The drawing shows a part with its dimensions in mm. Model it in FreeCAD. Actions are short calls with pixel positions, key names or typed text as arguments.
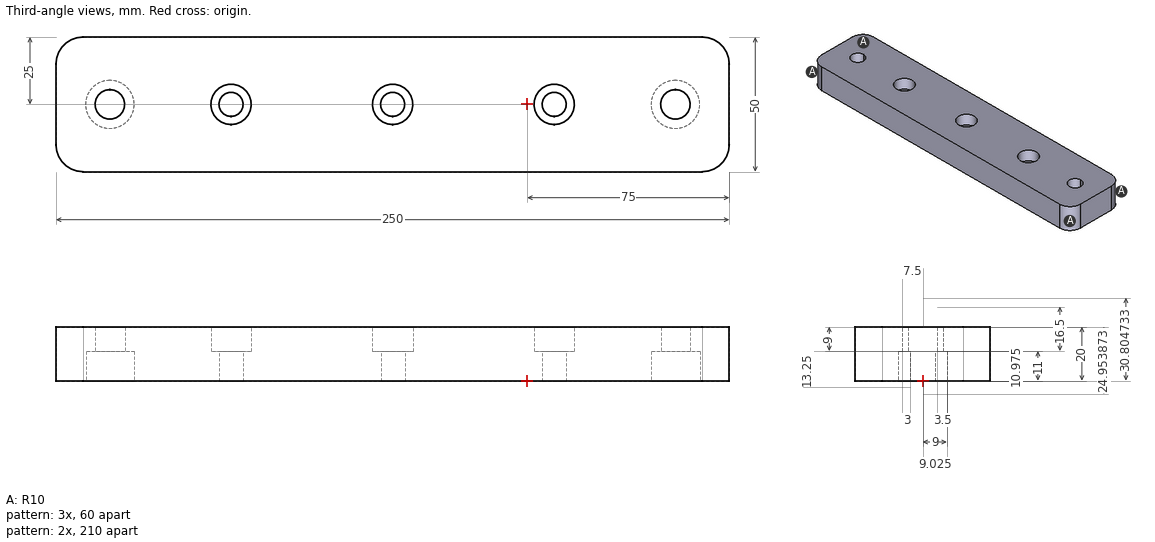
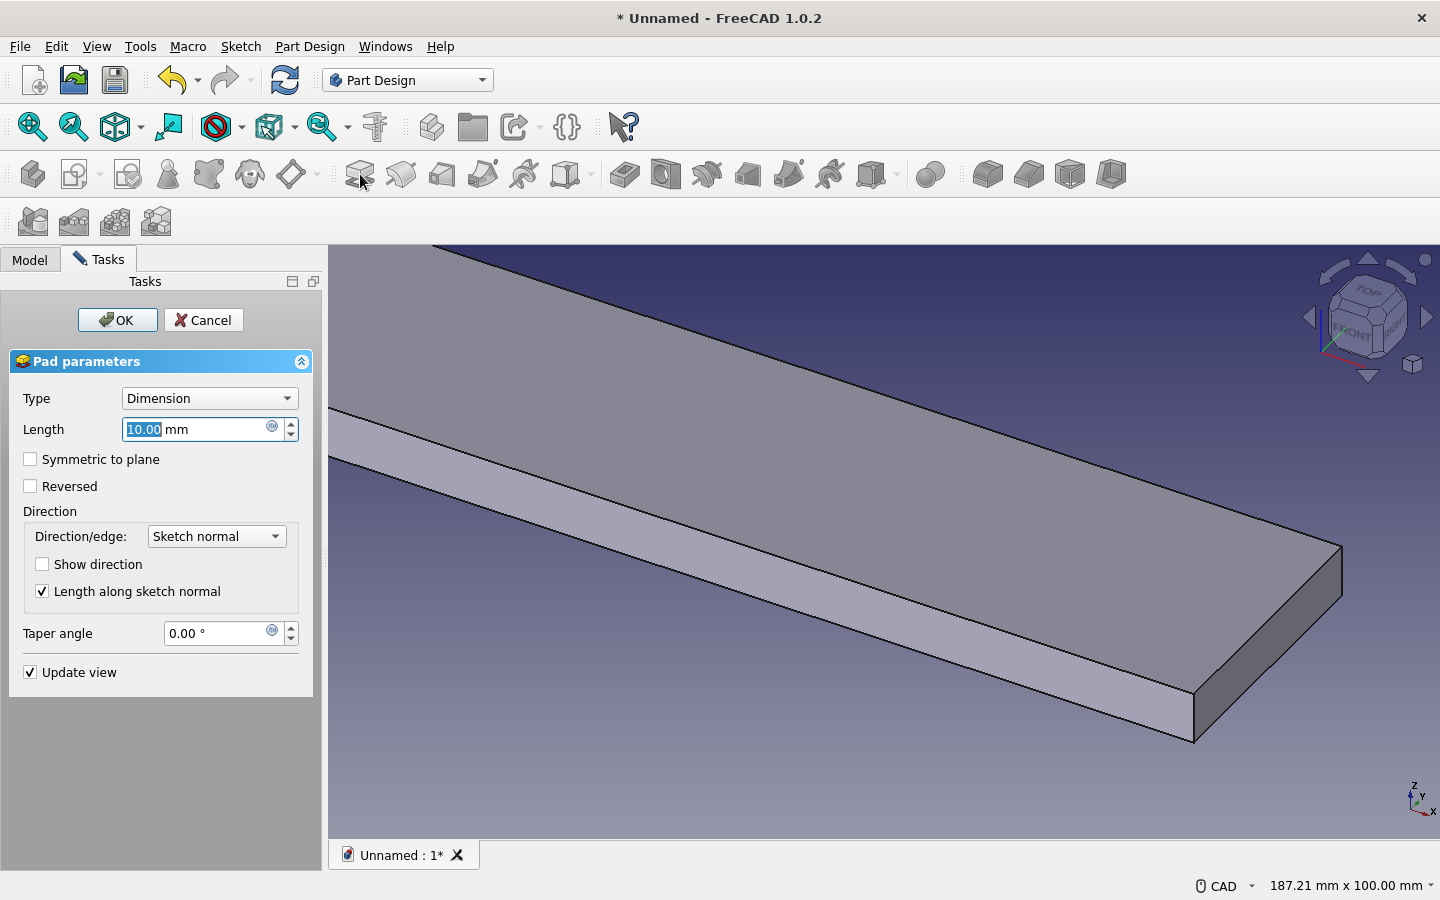
text(20)
key(Tab)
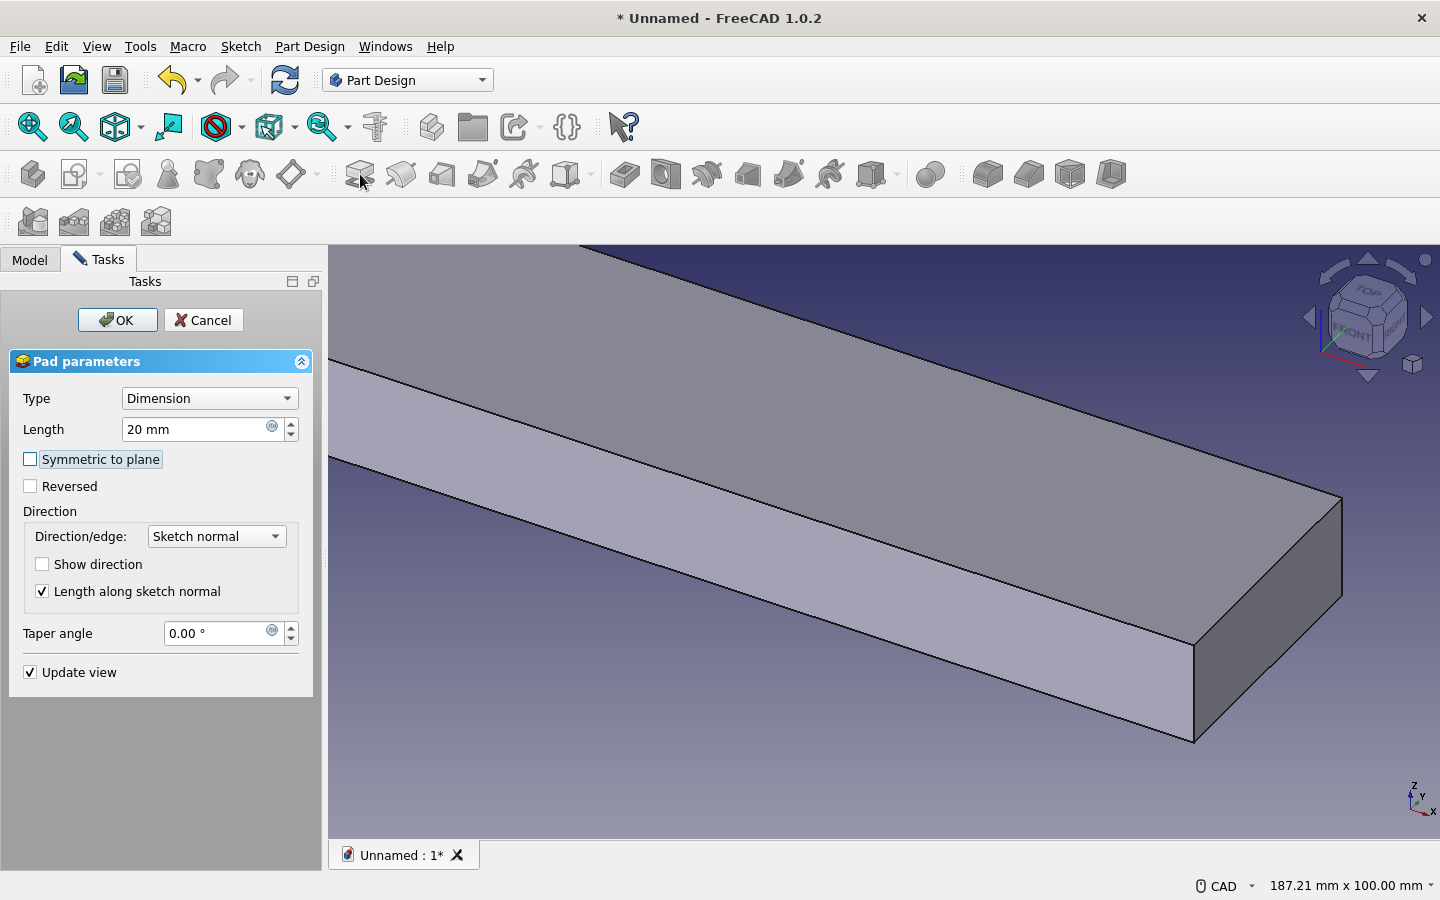
click(118, 320)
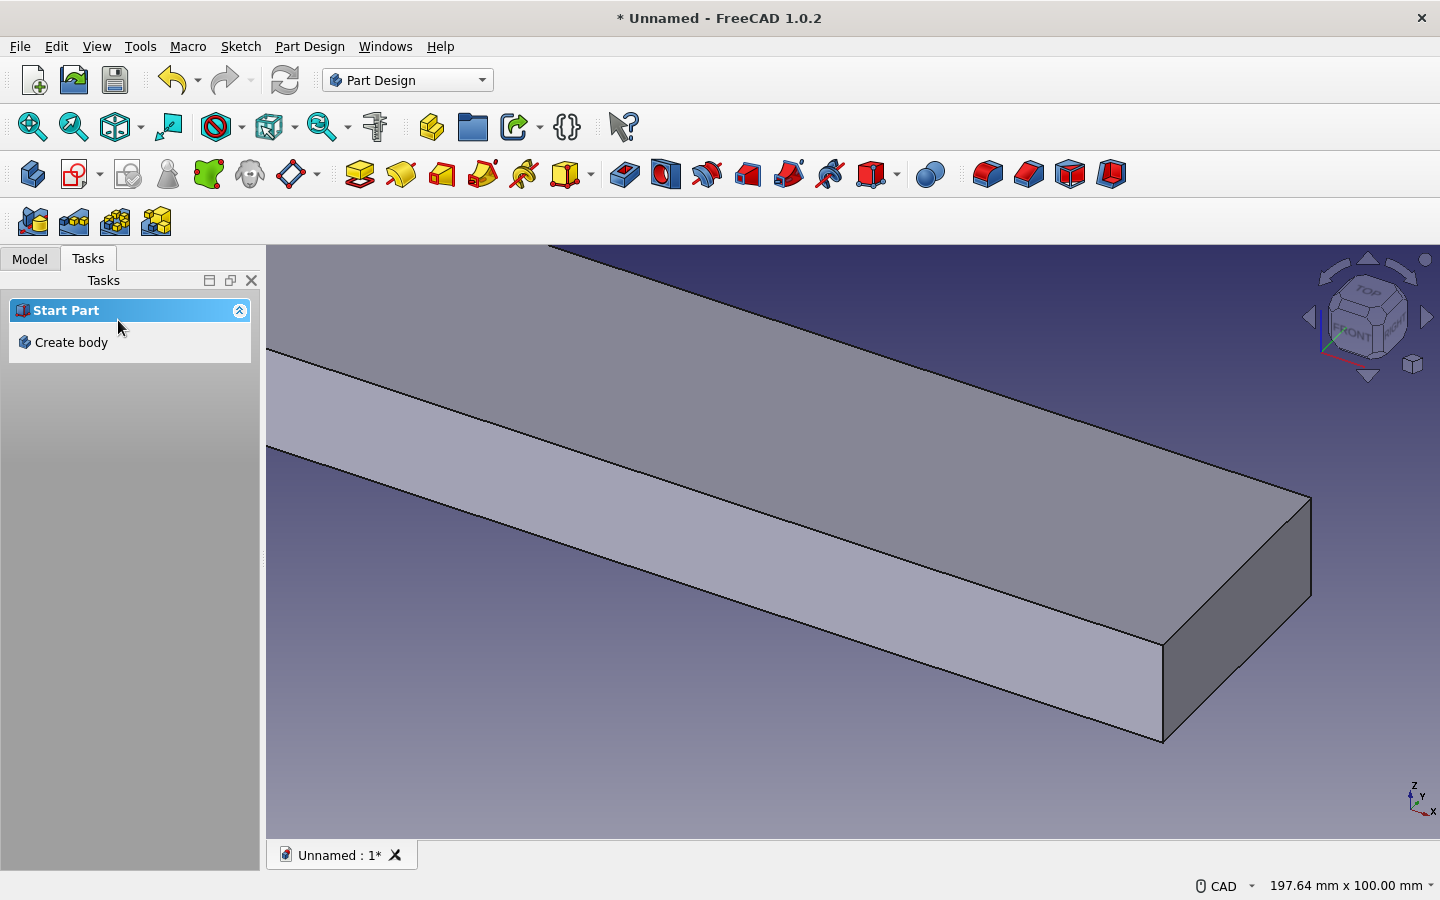
key(v)
key(f)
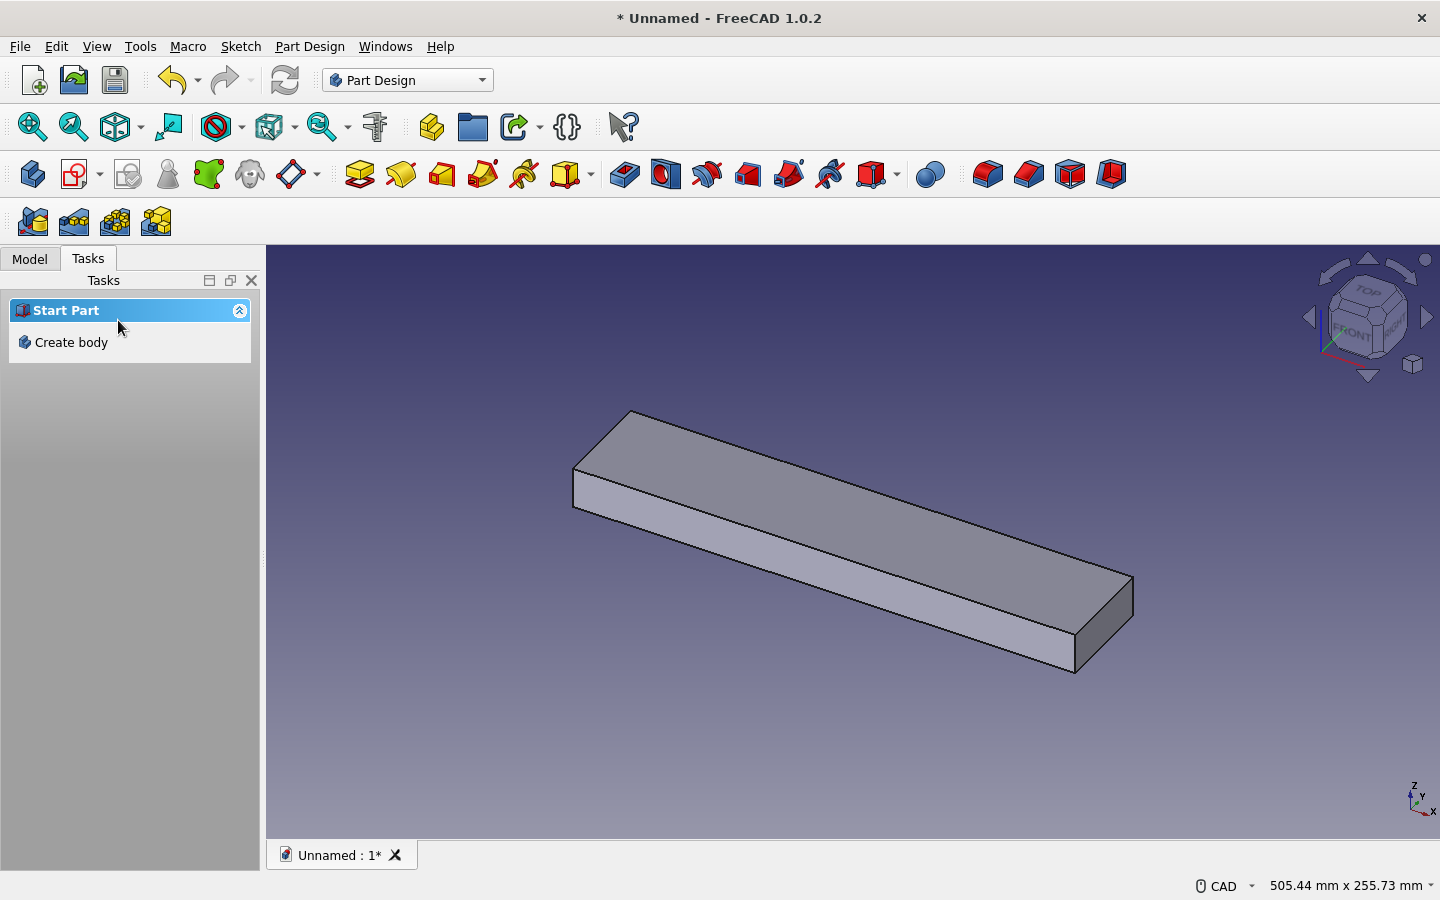
click(1075, 653)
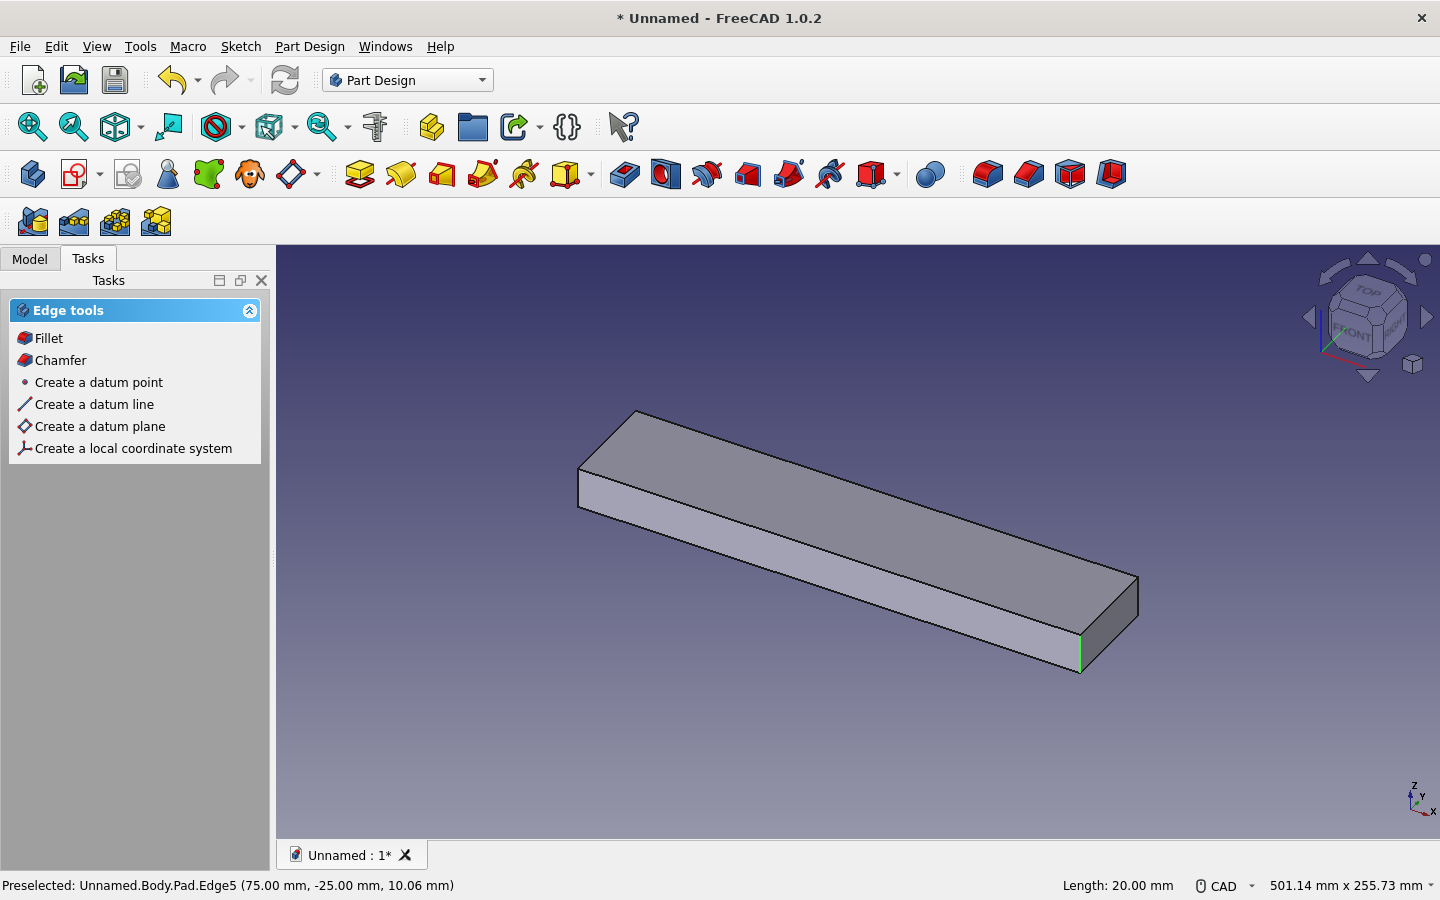
key(0)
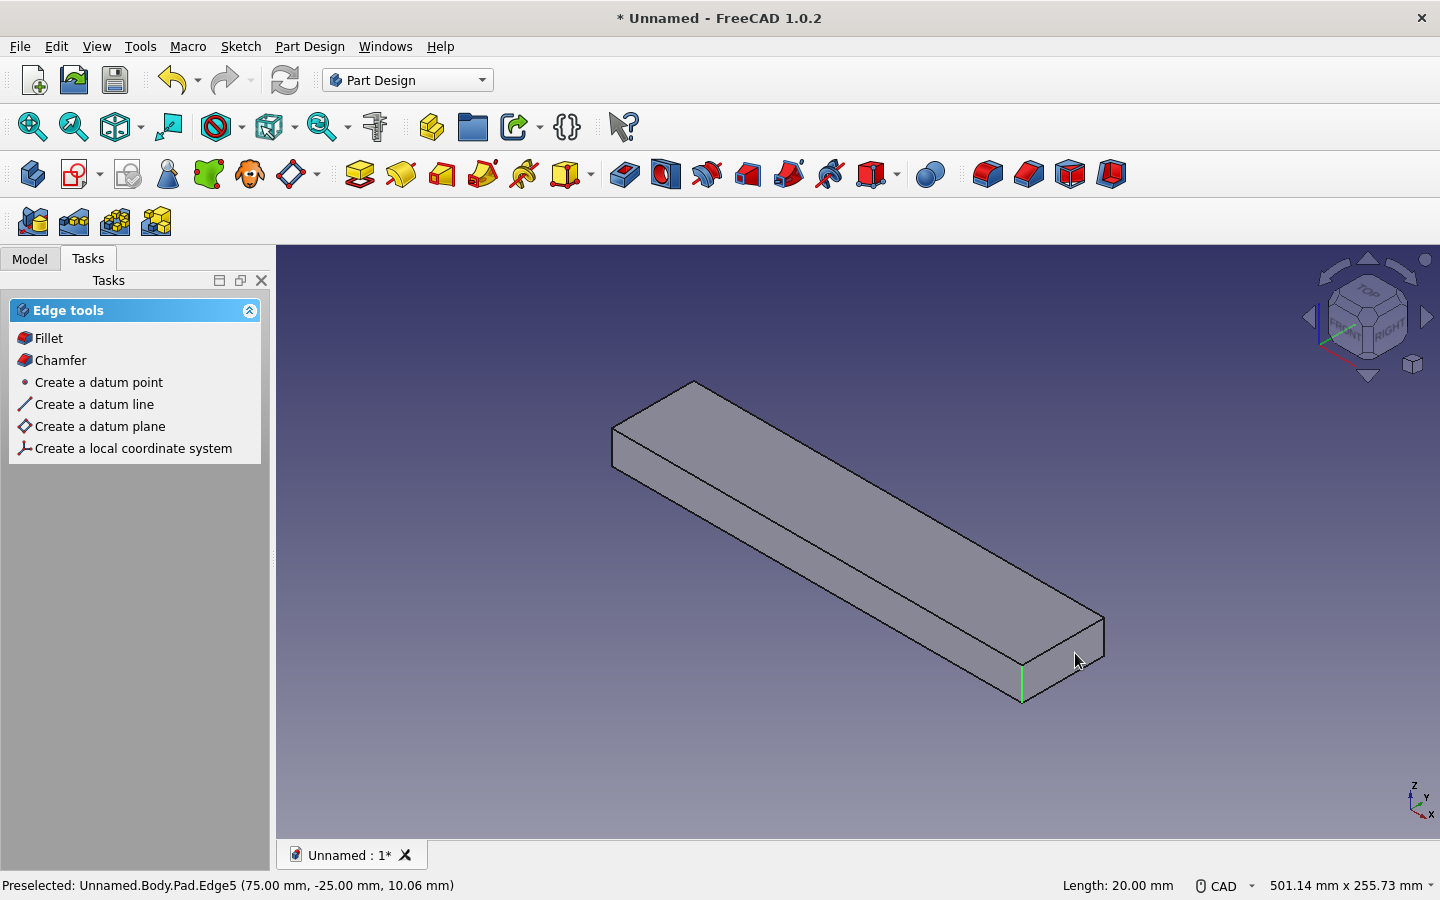
key(2)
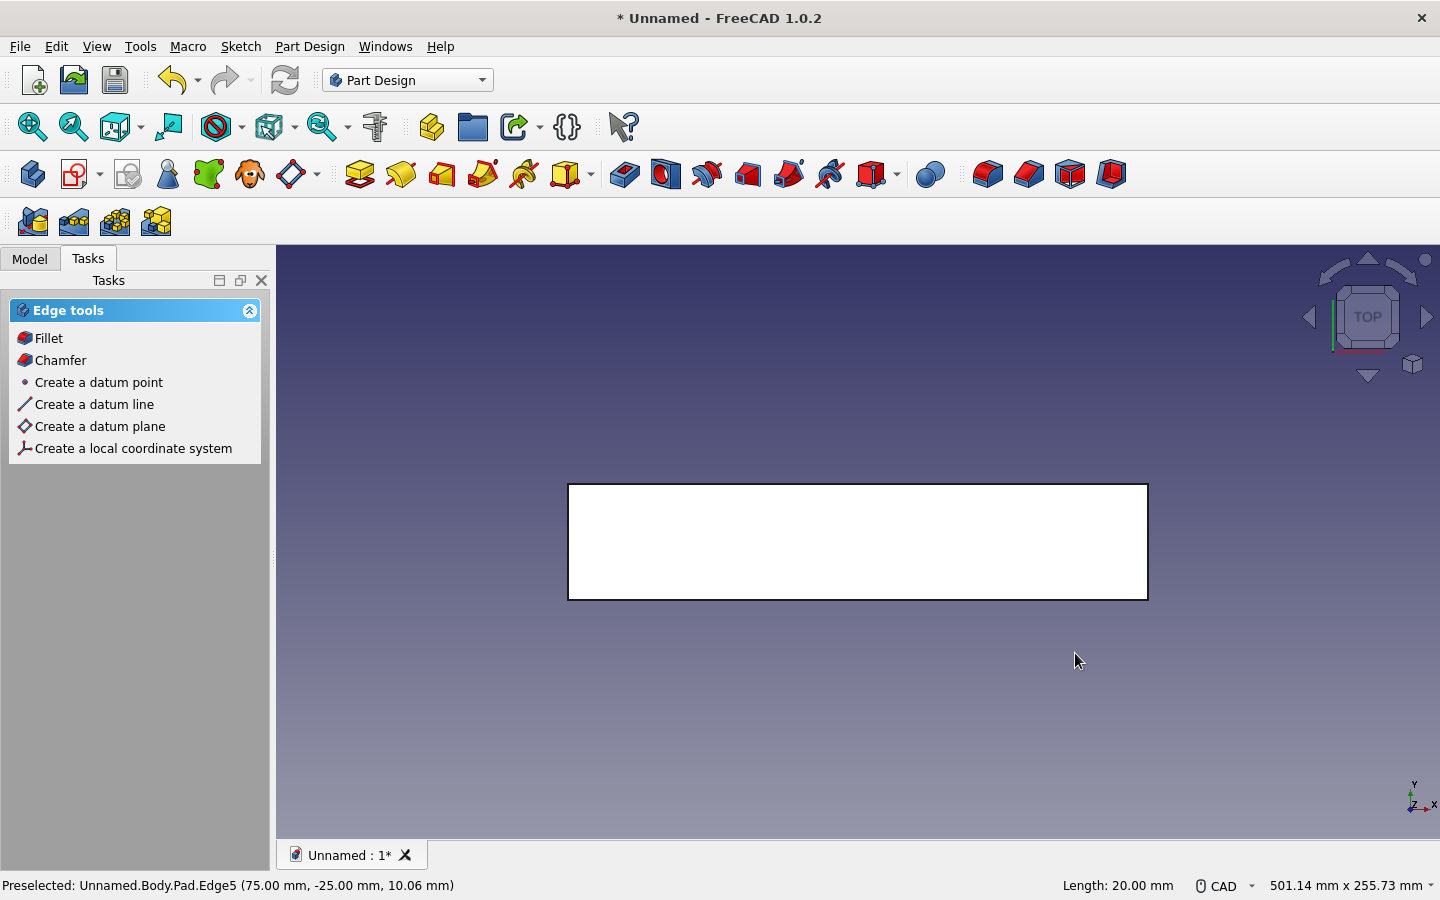
key(1)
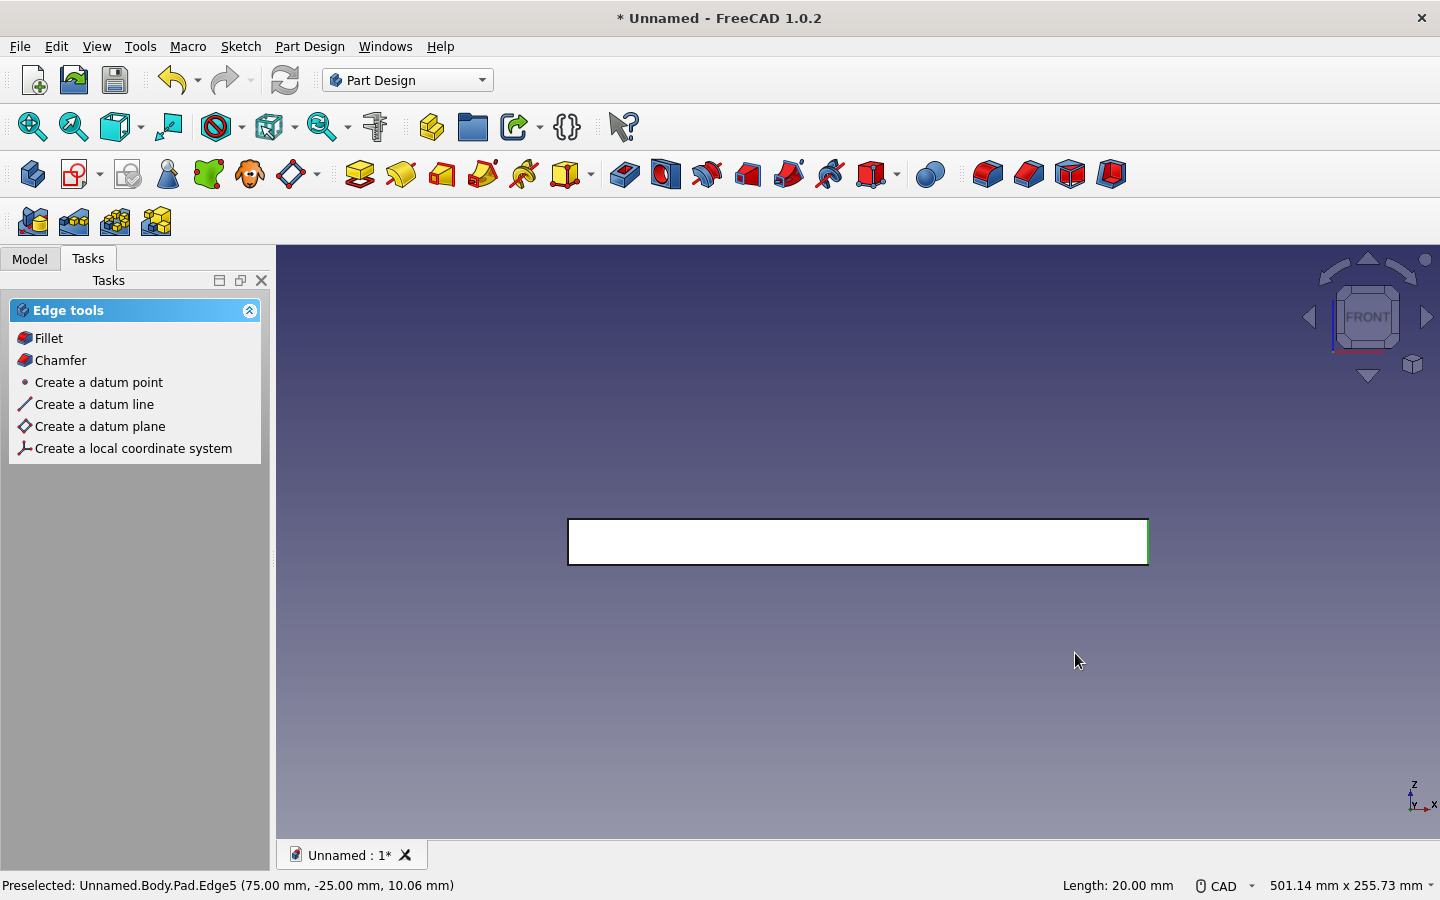
click(568, 541, ctrl)